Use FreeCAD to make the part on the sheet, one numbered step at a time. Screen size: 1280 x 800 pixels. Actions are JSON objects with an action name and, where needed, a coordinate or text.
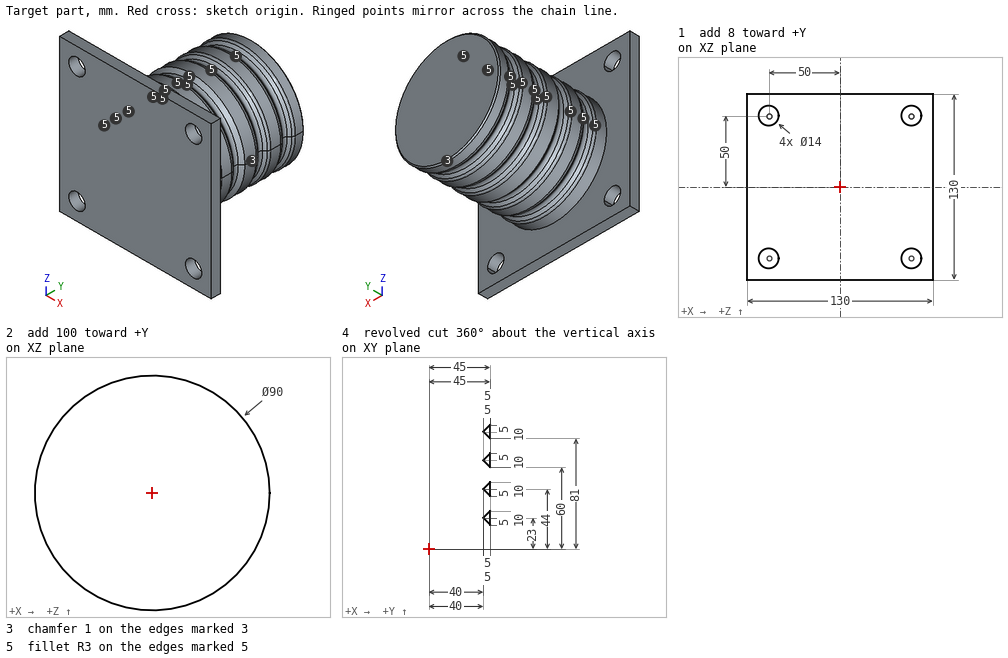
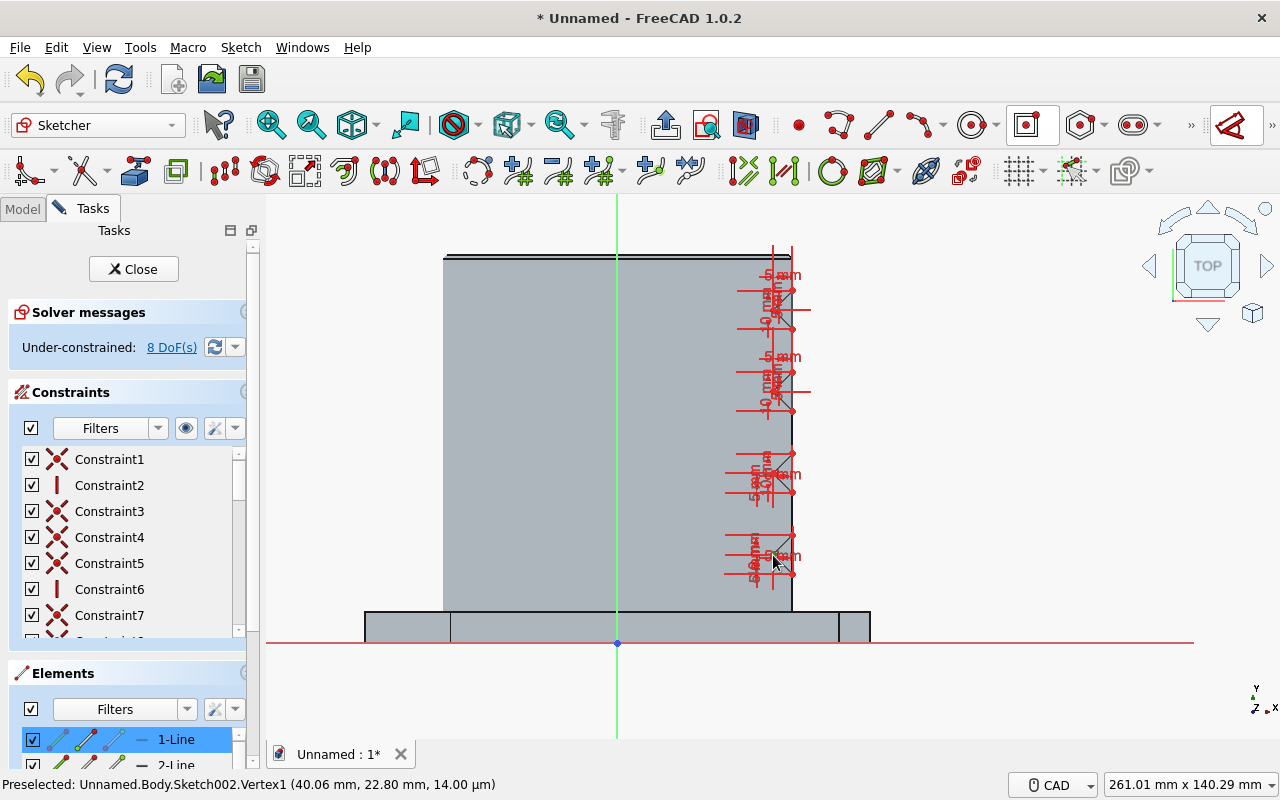
{"action": "key", "text": "l"}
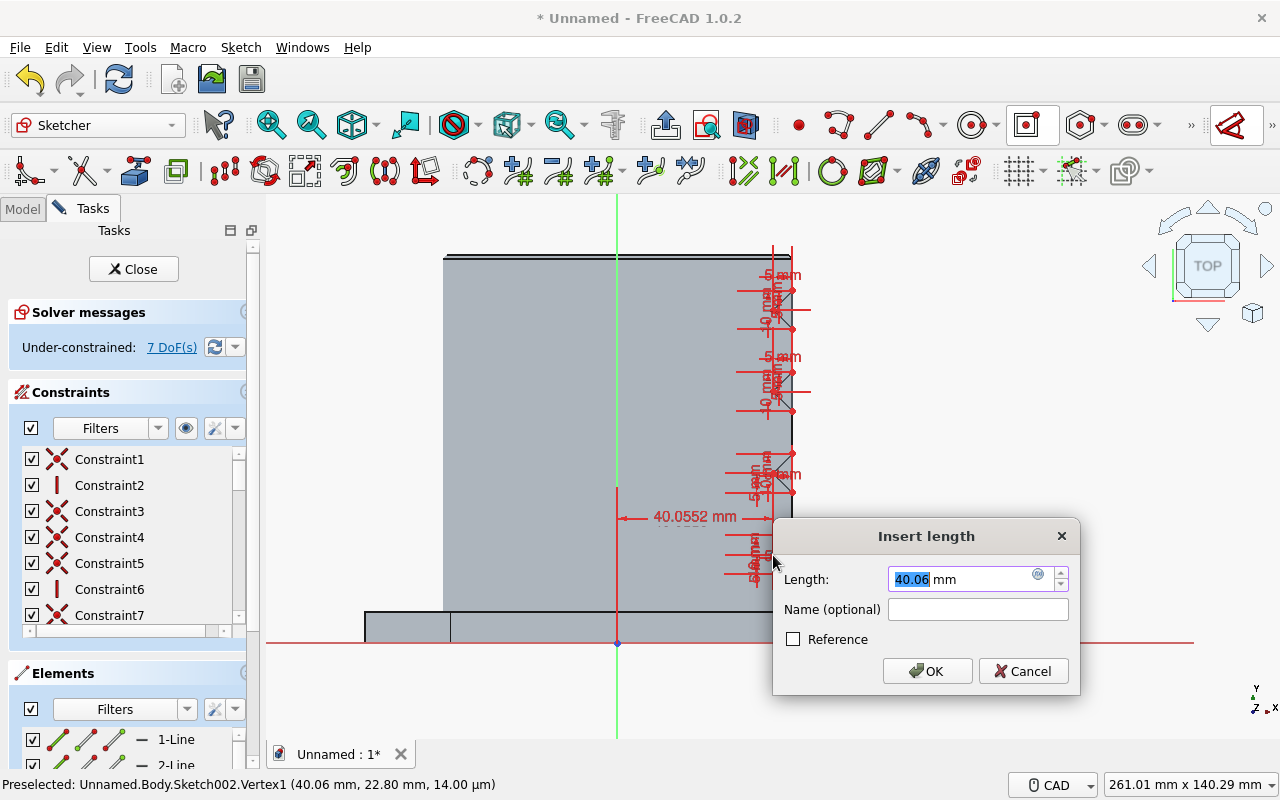
{"action": "type", "text": "40"}
{"action": "key", "text": "Return"}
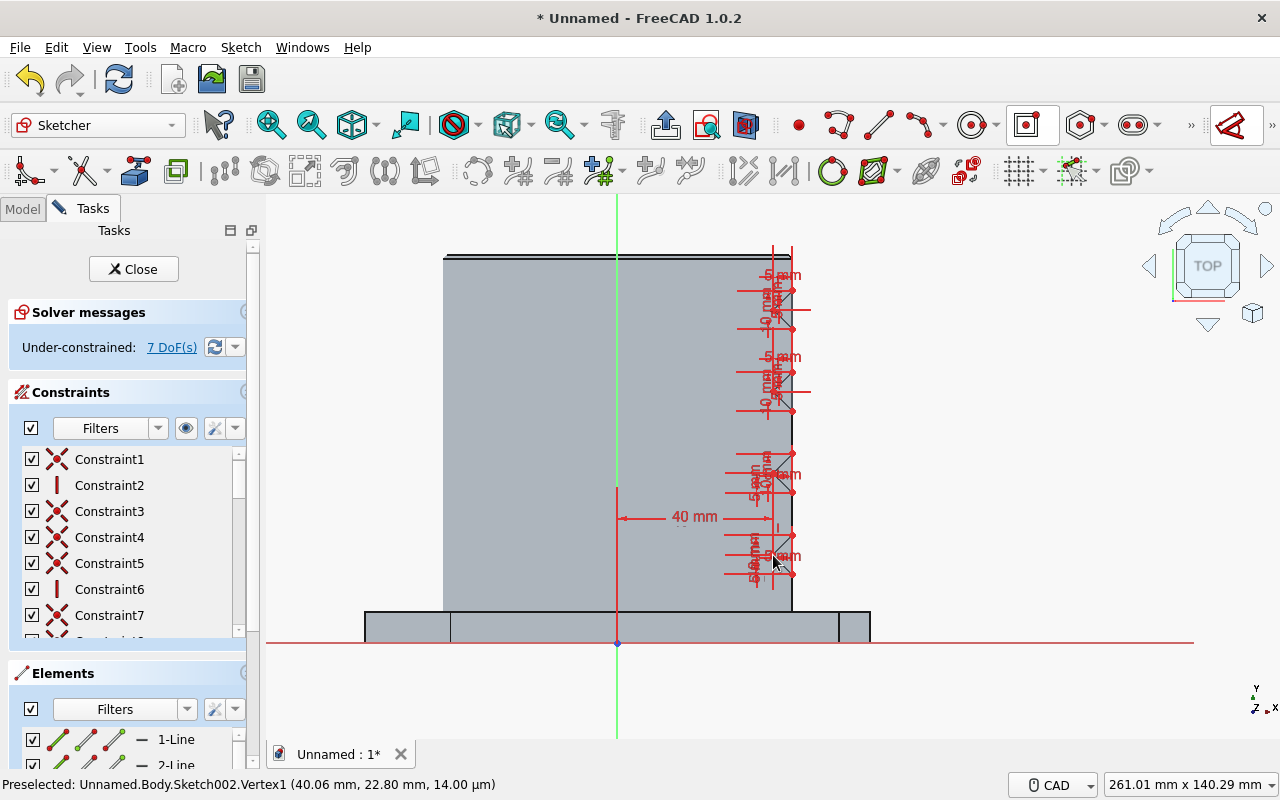
{"action": "left_click", "coordinate": [773, 555]}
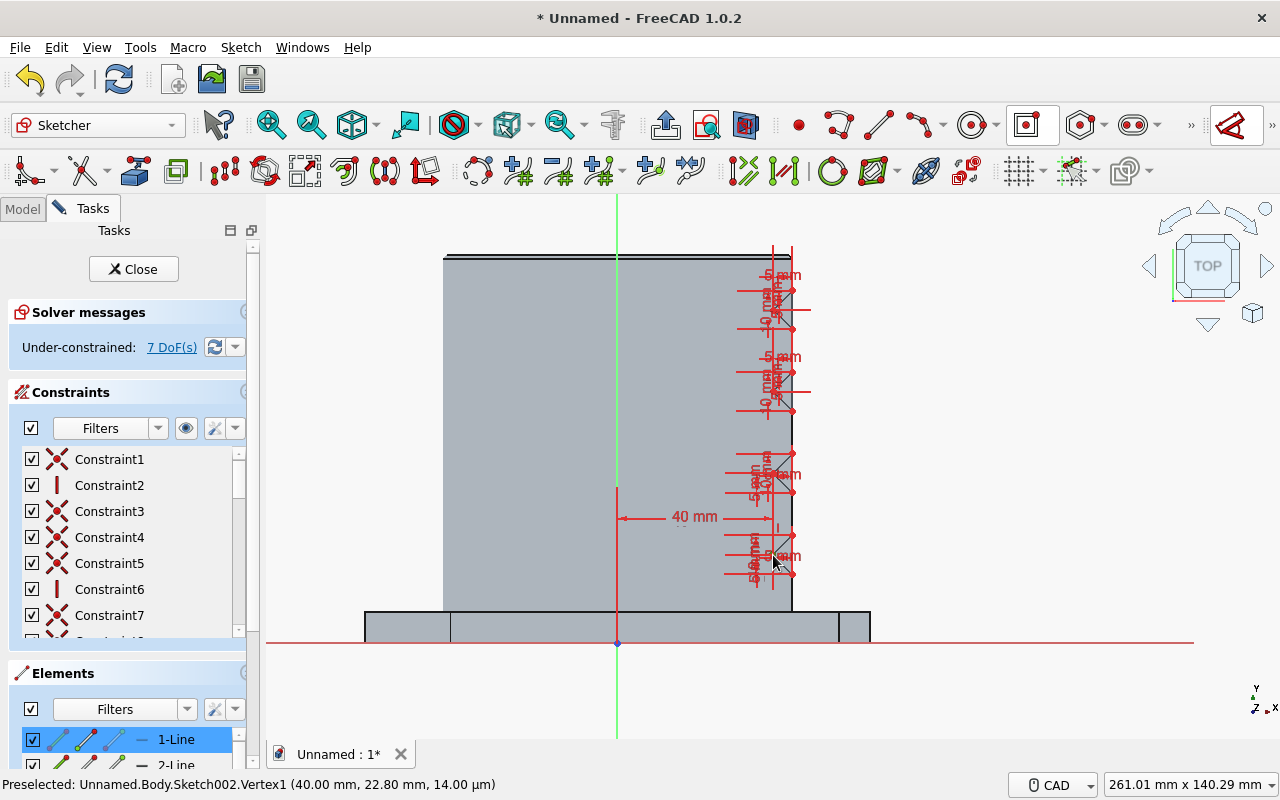
{"action": "key", "text": "i"}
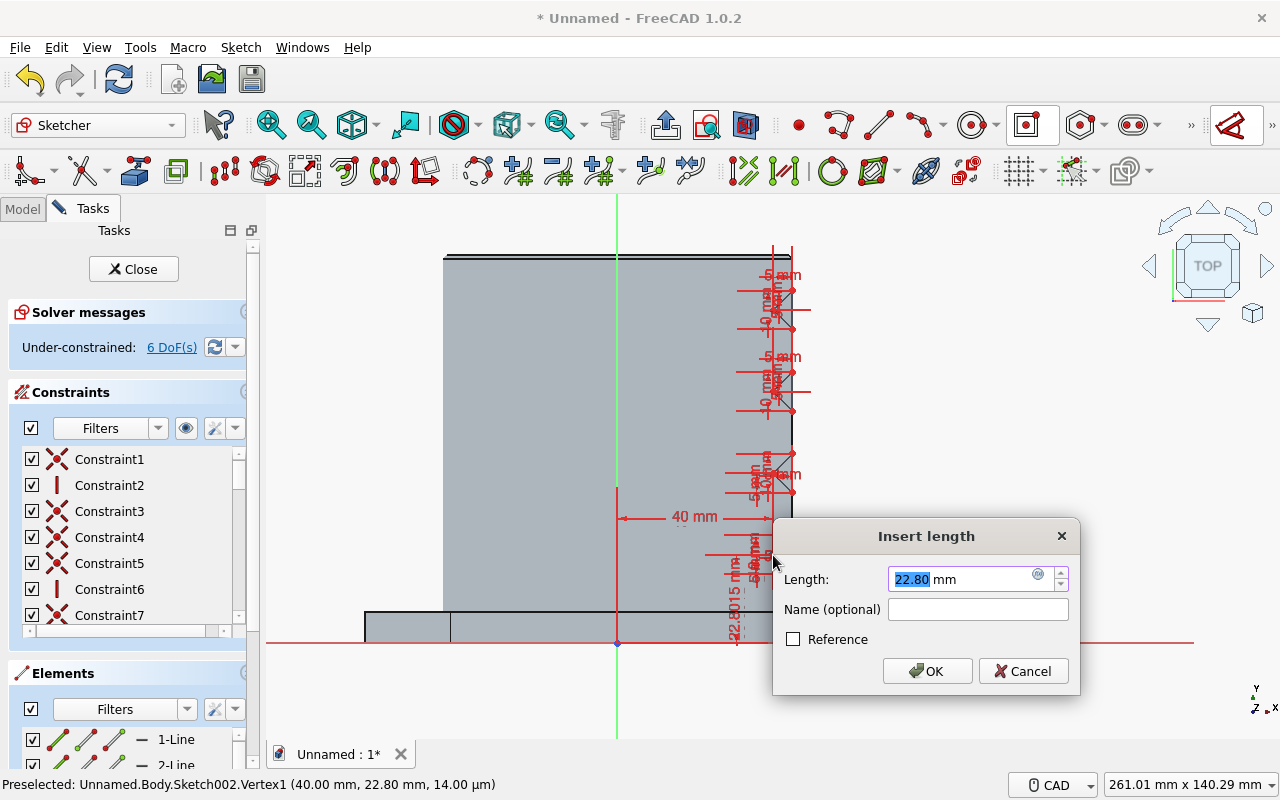
{"action": "type", "text": "23"}
{"action": "key", "text": "Return"}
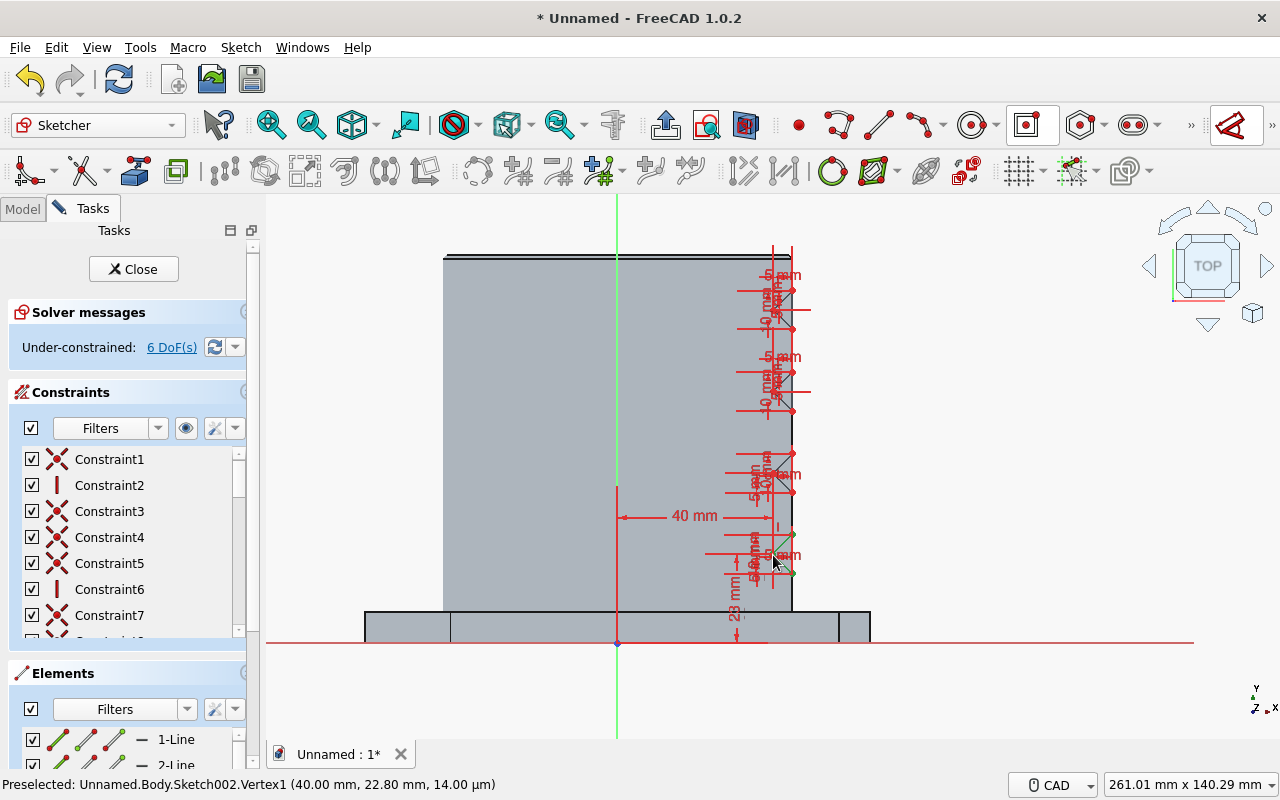
{"action": "left_click", "coordinate": [773, 473]}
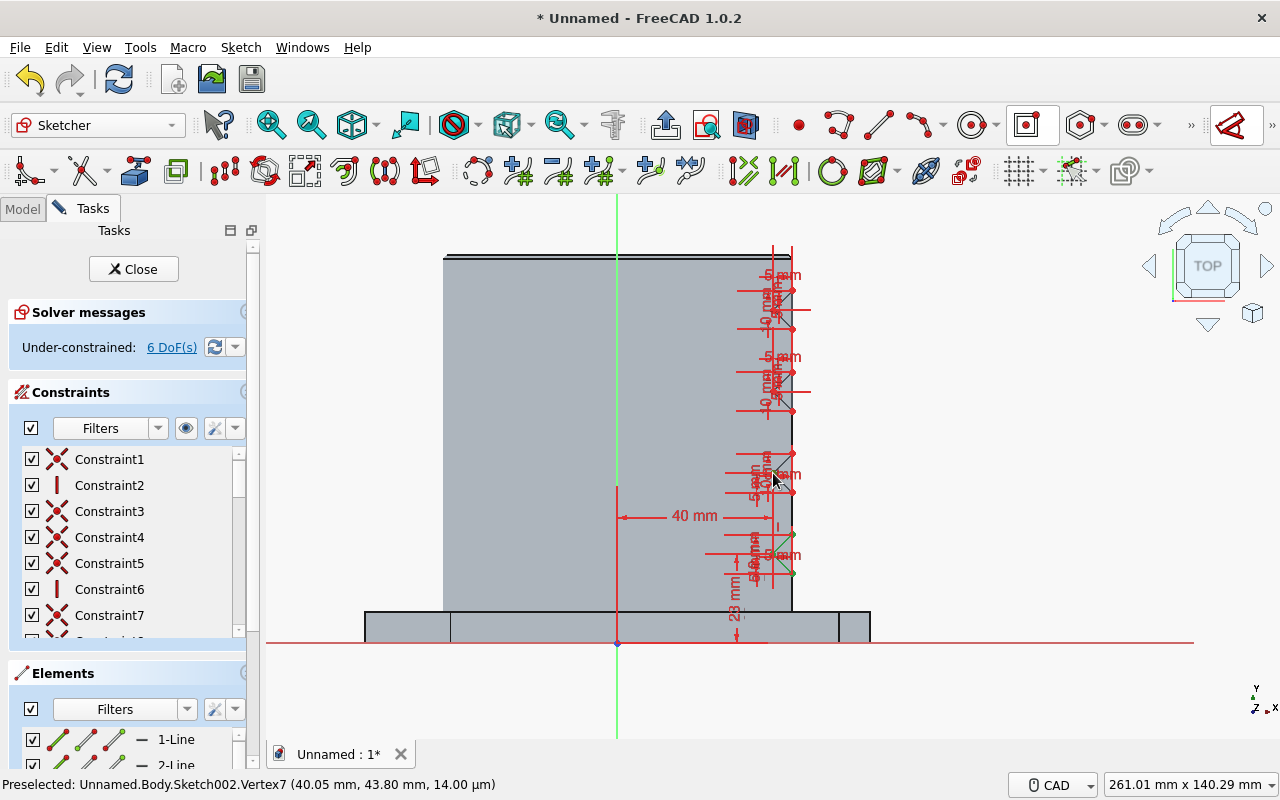
{"action": "left_click", "coordinate": [1258, 126]}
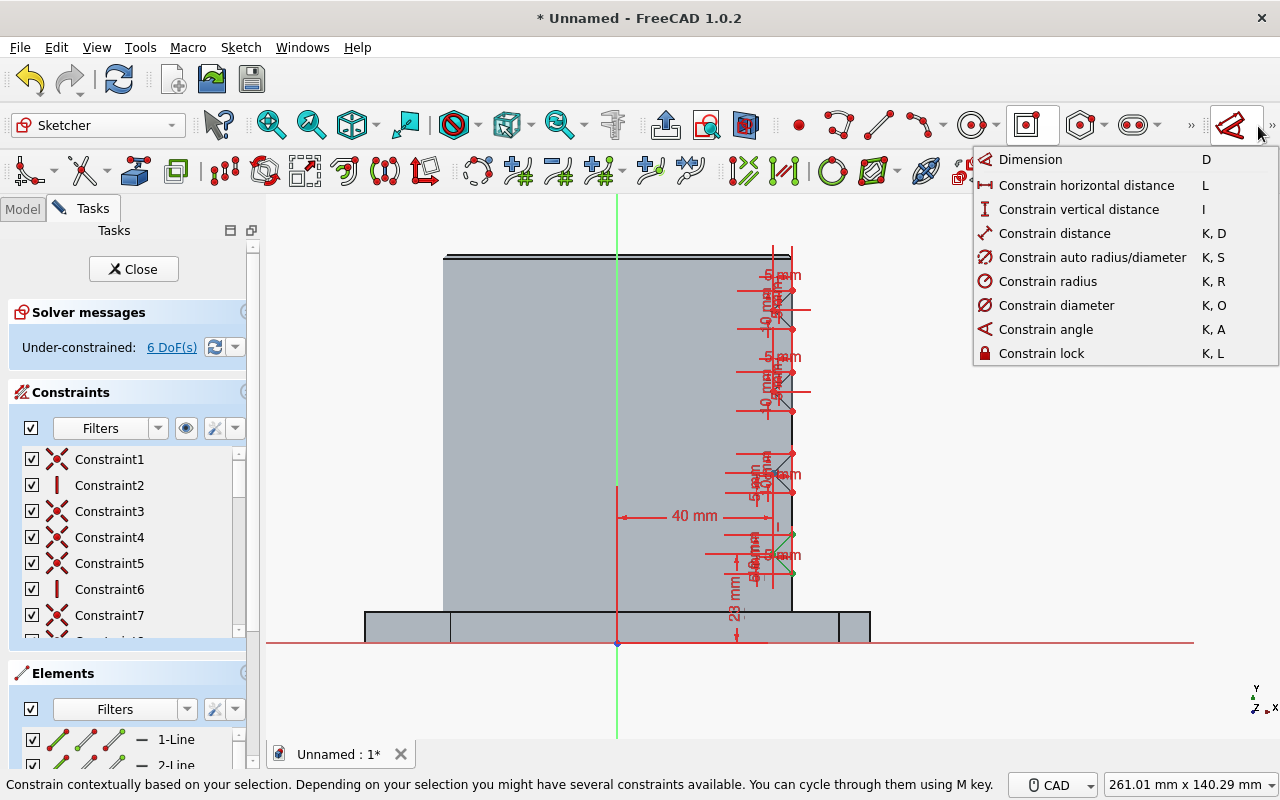
{"action": "left_click", "coordinate": [1126, 185]}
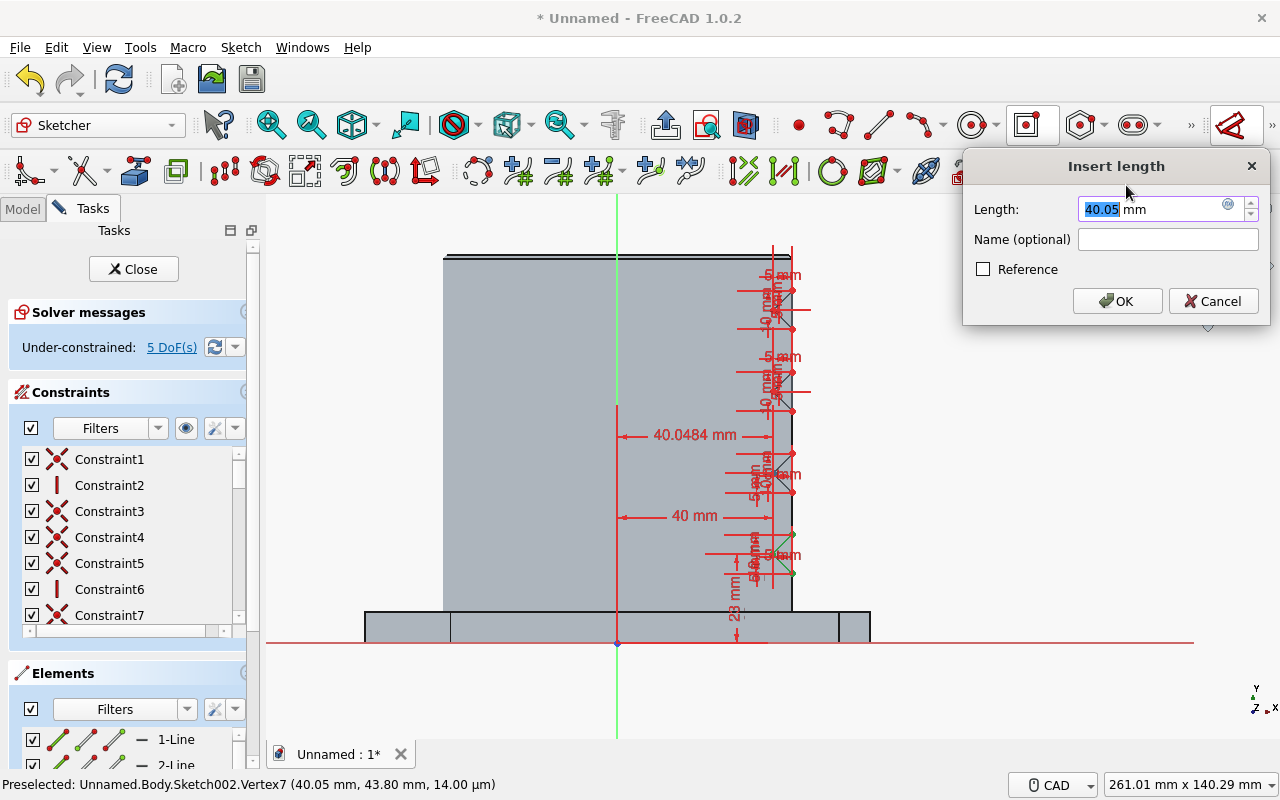
{"action": "type", "text": "40"}
{"action": "key", "text": "Return"}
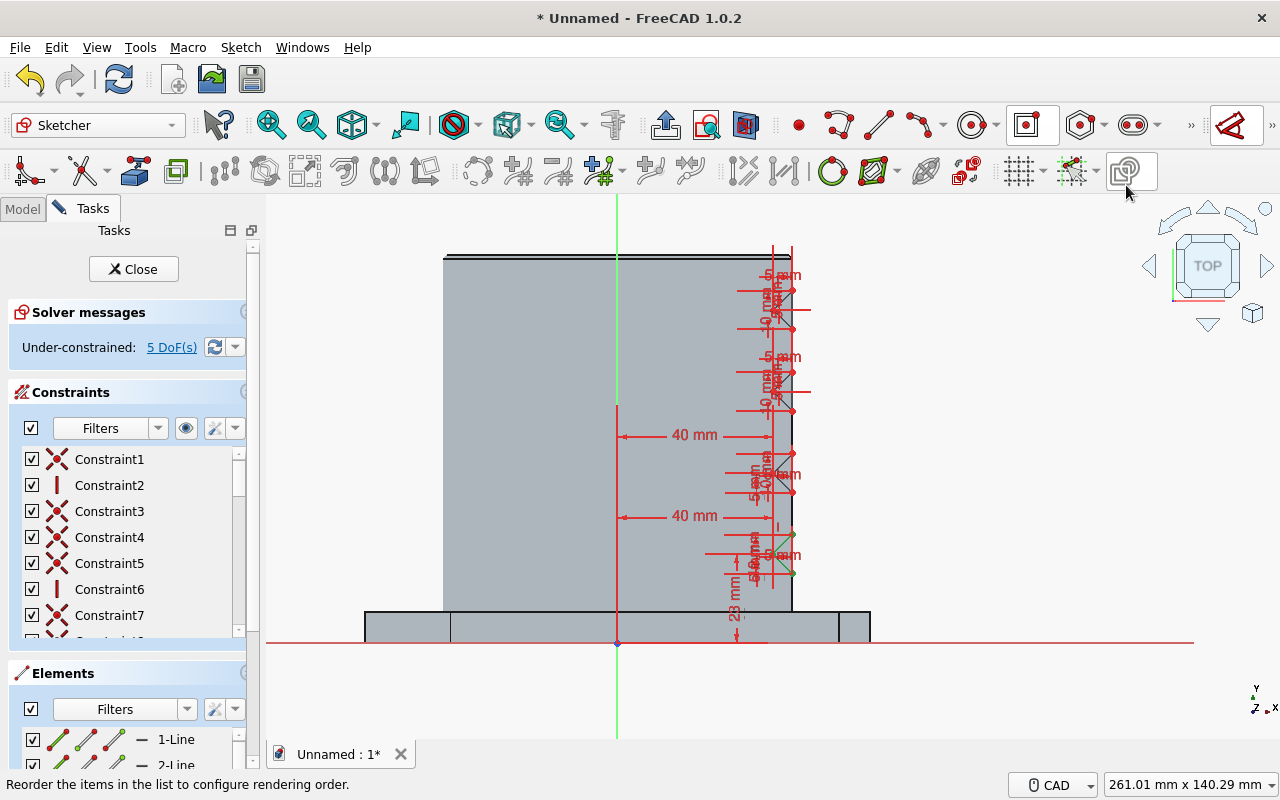
{"action": "left_click", "coordinate": [773, 473]}